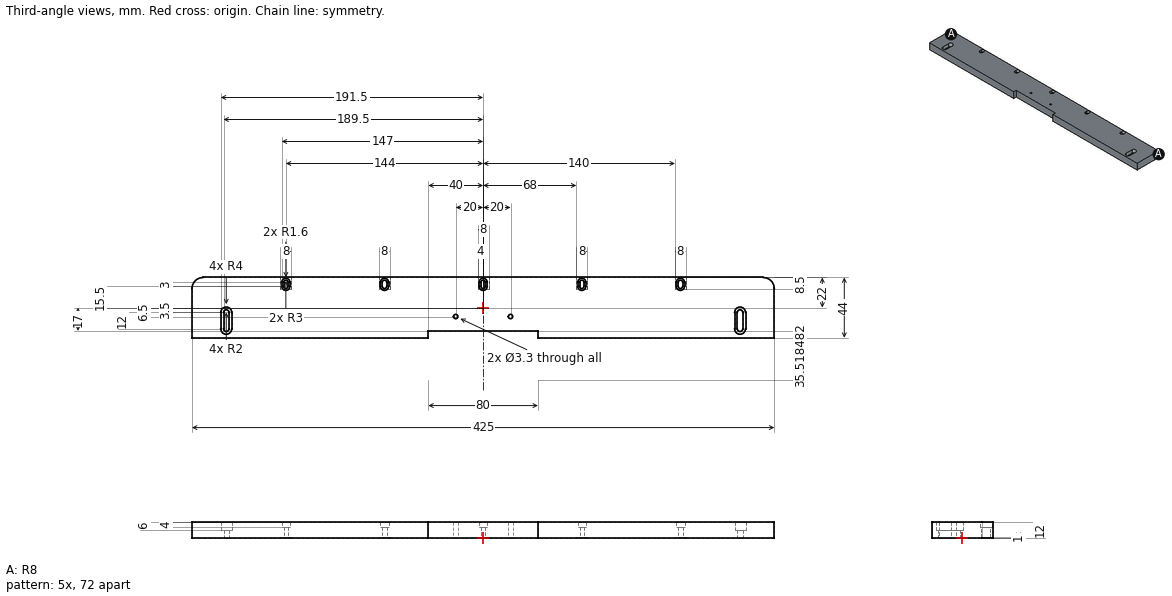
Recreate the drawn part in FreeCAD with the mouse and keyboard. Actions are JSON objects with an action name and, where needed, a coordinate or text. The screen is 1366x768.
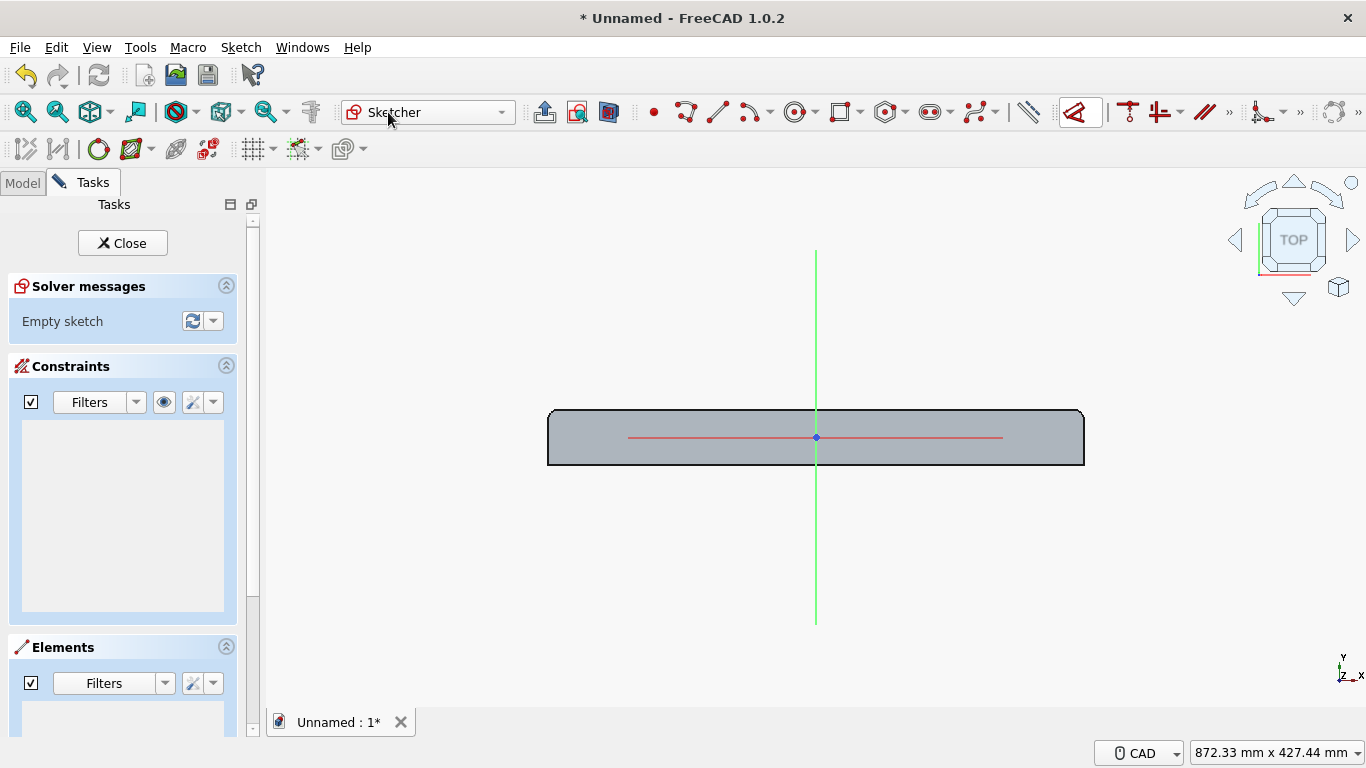
{"action": "left_click", "coordinate": [930, 112]}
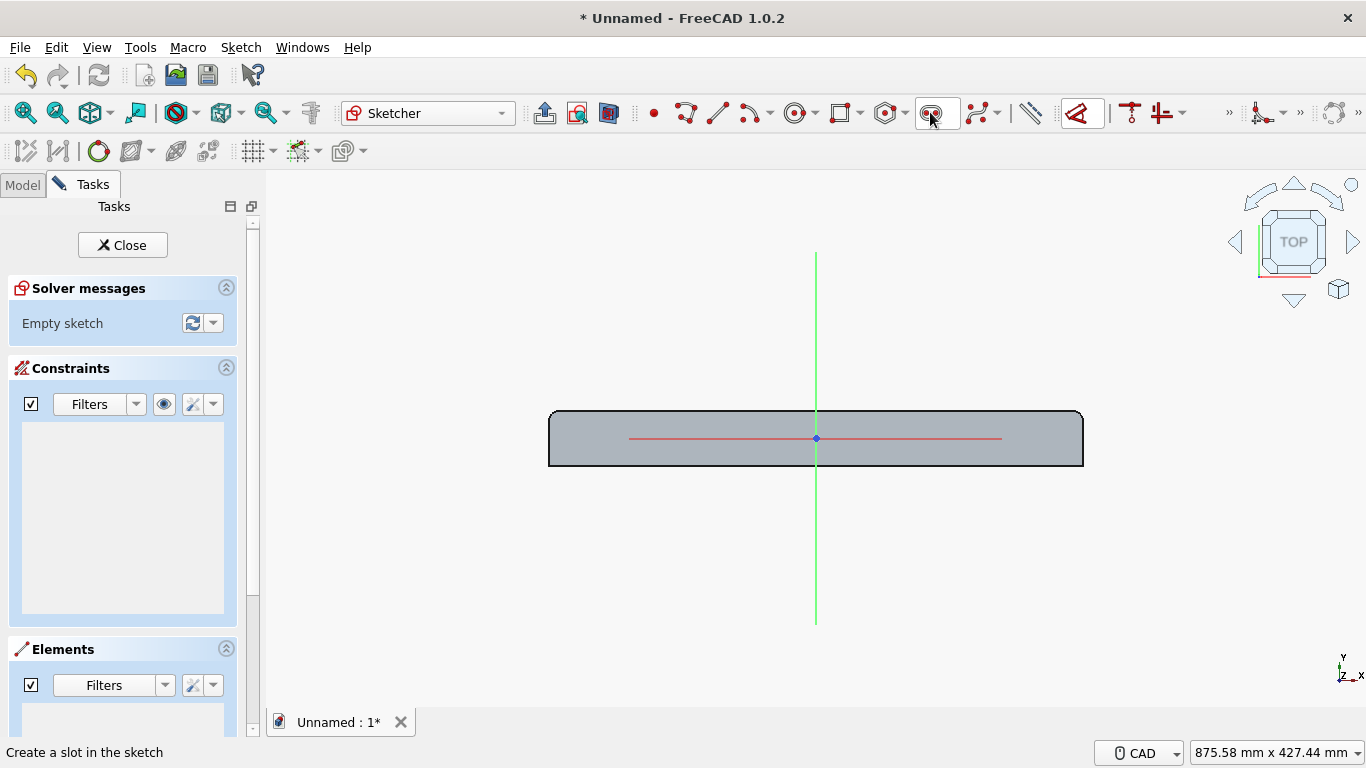
{"action": "scroll", "coordinate": [580, 458], "scroll_direction": "up", "scroll_amount": 8}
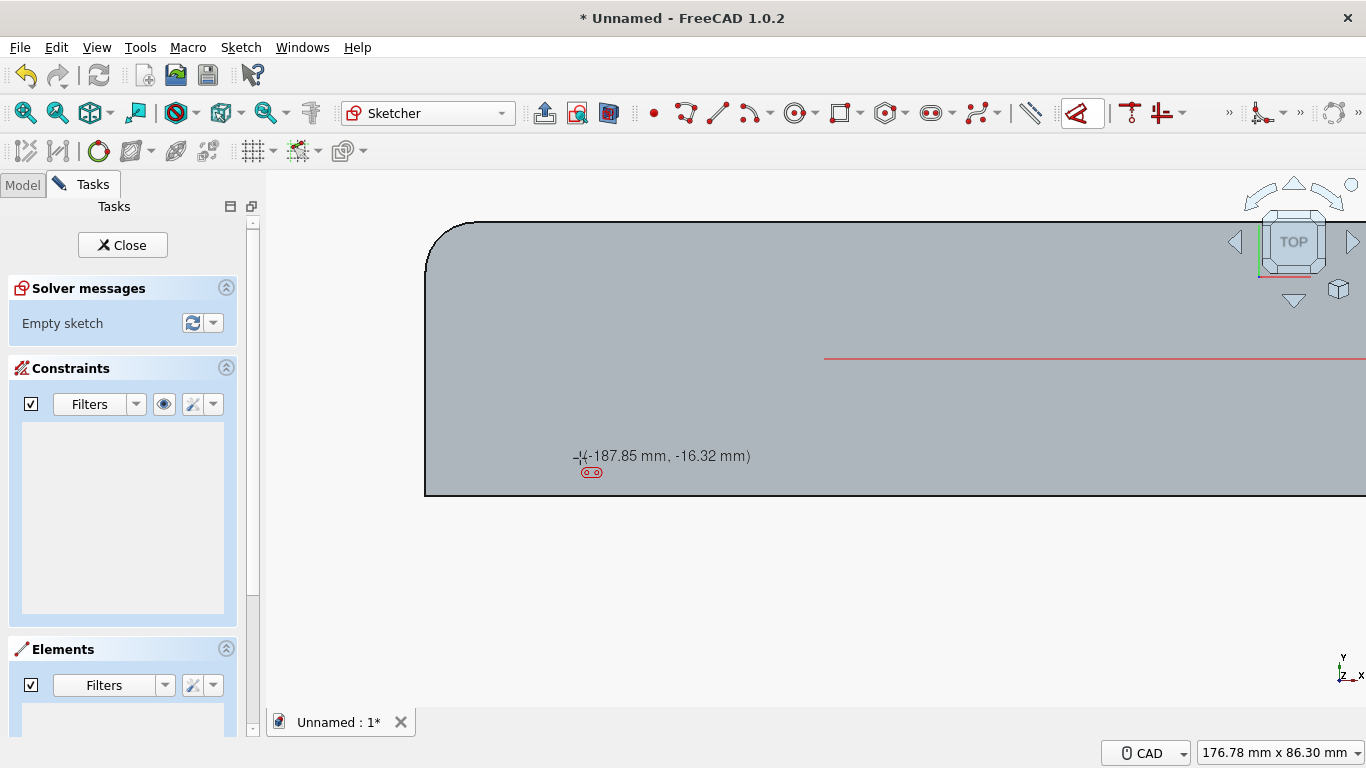
{"action": "scroll", "coordinate": [420, 445], "scroll_direction": "down", "scroll_amount": 7}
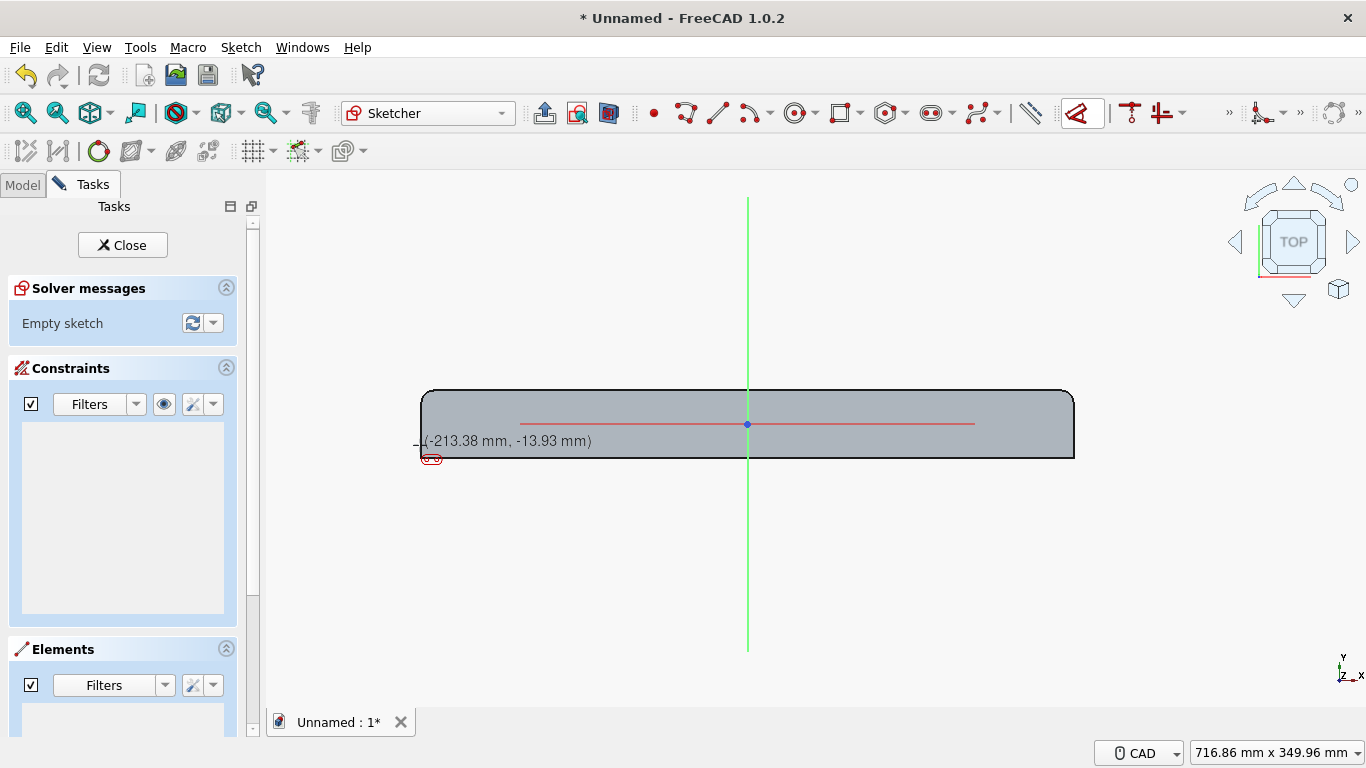
{"action": "left_click", "coordinate": [460, 448]}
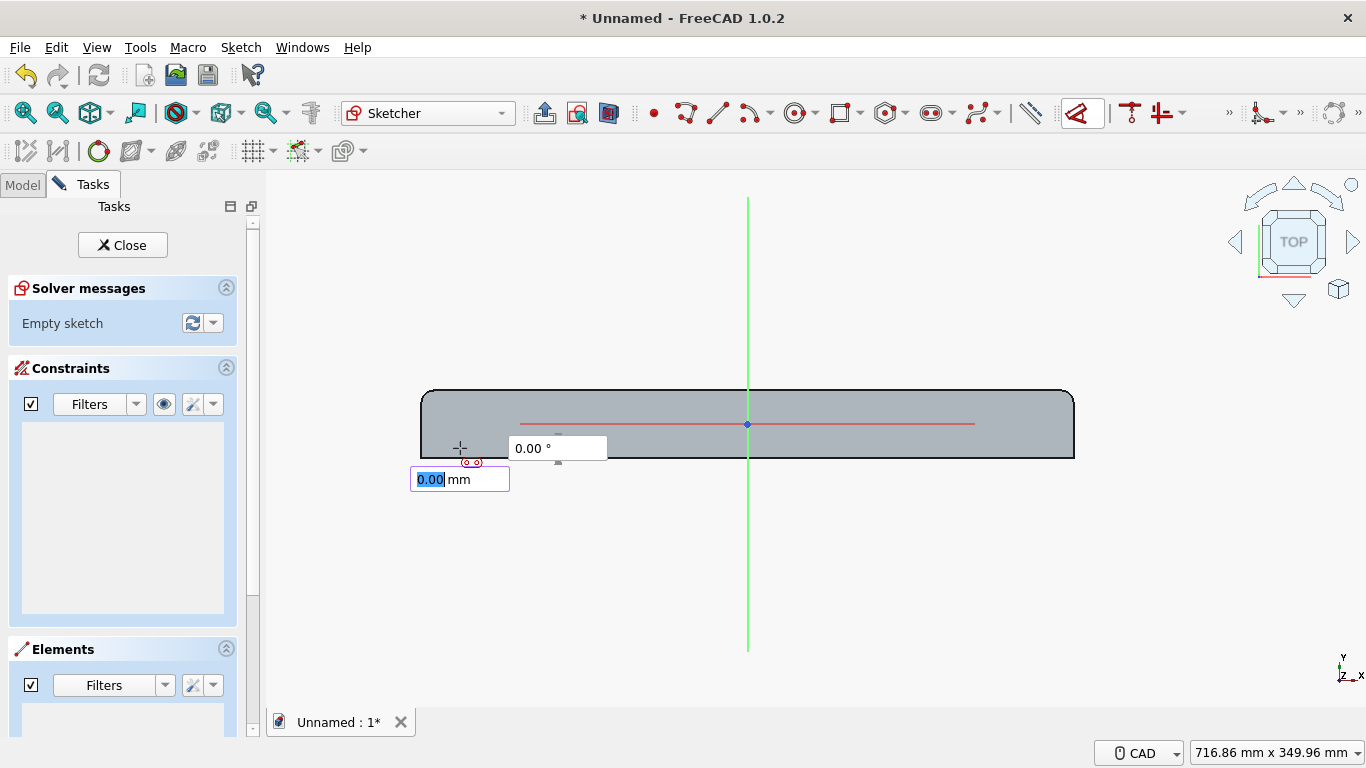
{"action": "scroll", "coordinate": [460, 430], "scroll_direction": "up", "scroll_amount": 6}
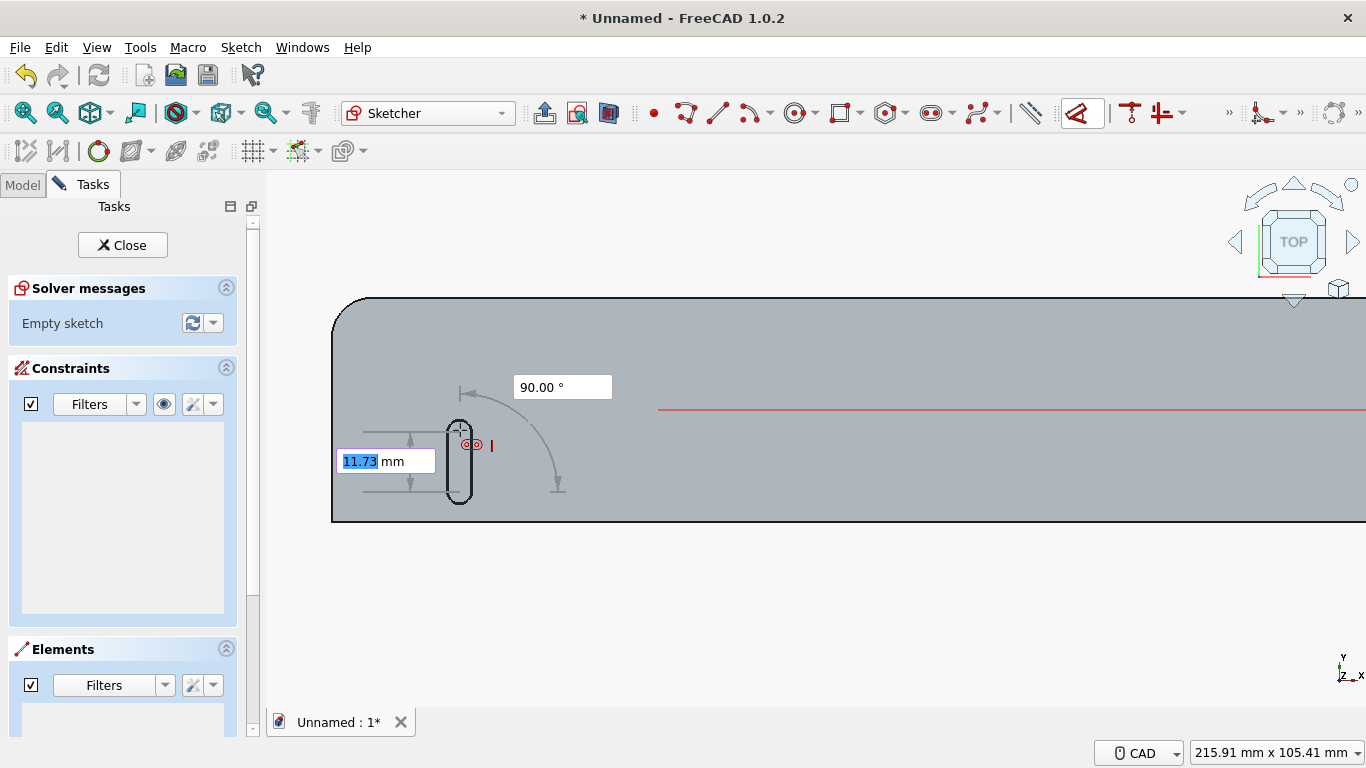
{"action": "left_click", "coordinate": [460, 428]}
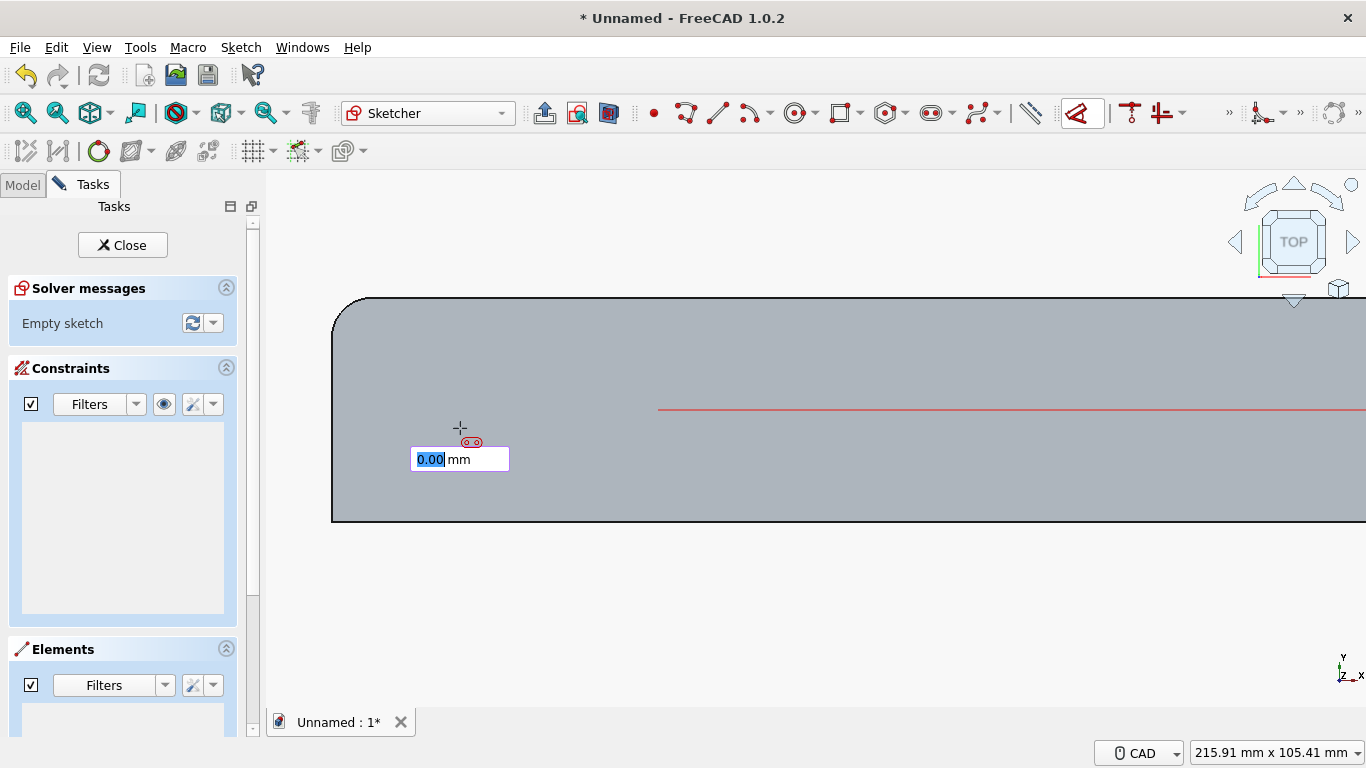
{"action": "left_click", "coordinate": [479, 458]}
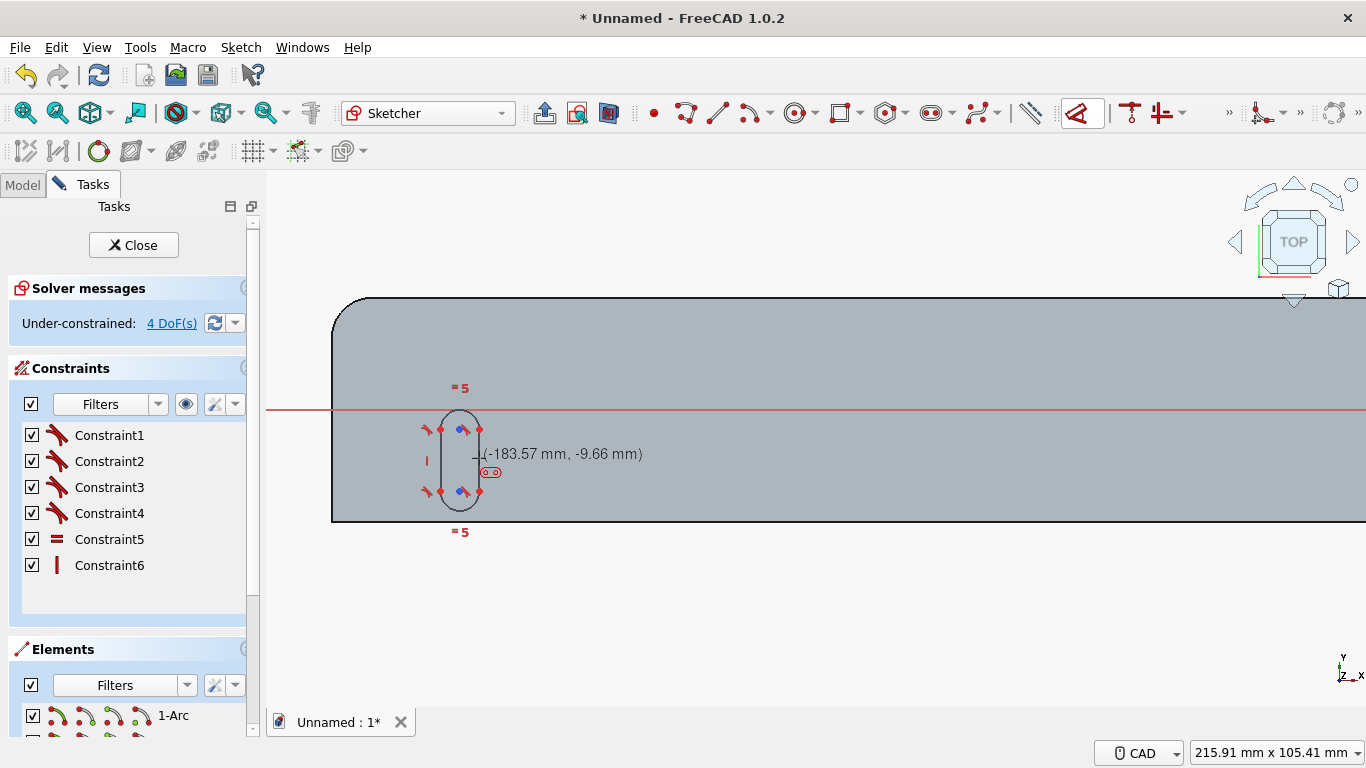
{"action": "scroll", "coordinate": [460, 430], "scroll_direction": "down", "scroll_amount": 6}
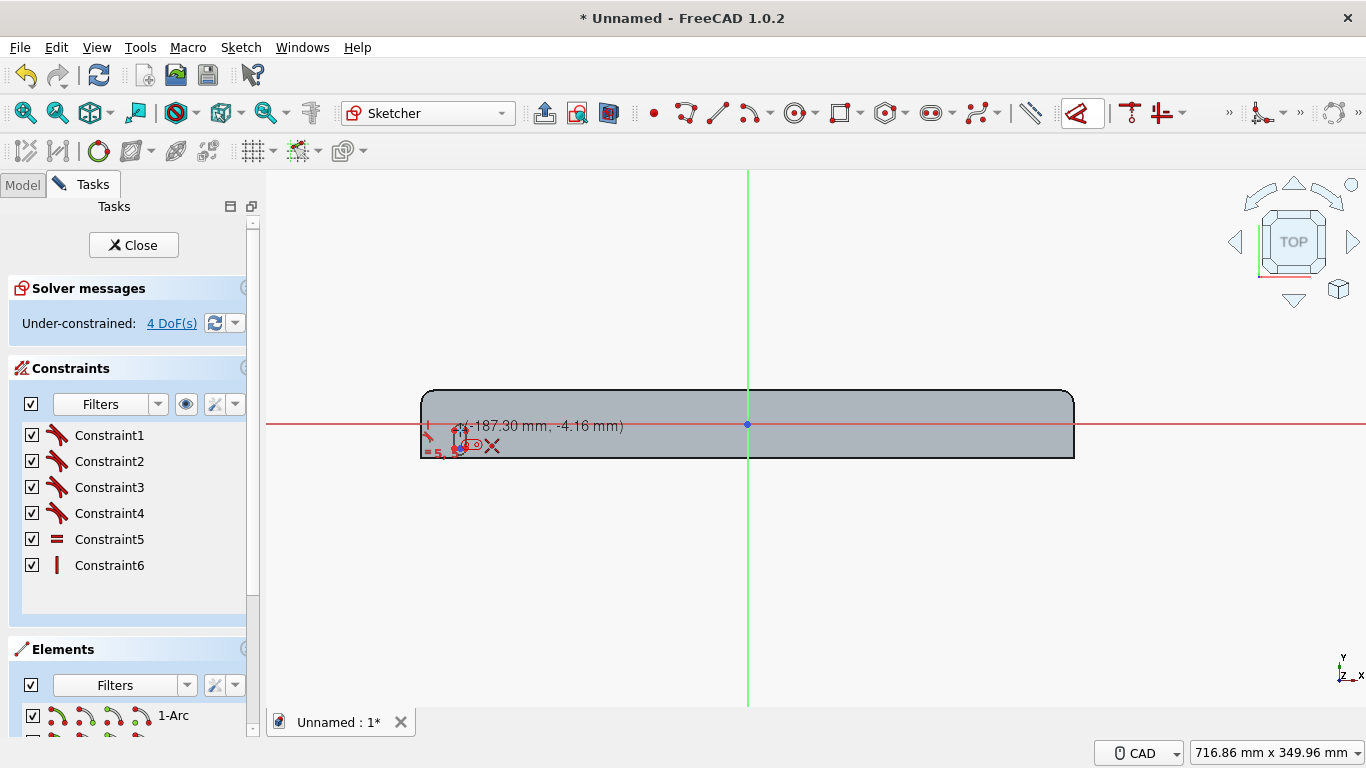
{"action": "scroll", "coordinate": [1035, 448], "scroll_direction": "up", "scroll_amount": 7}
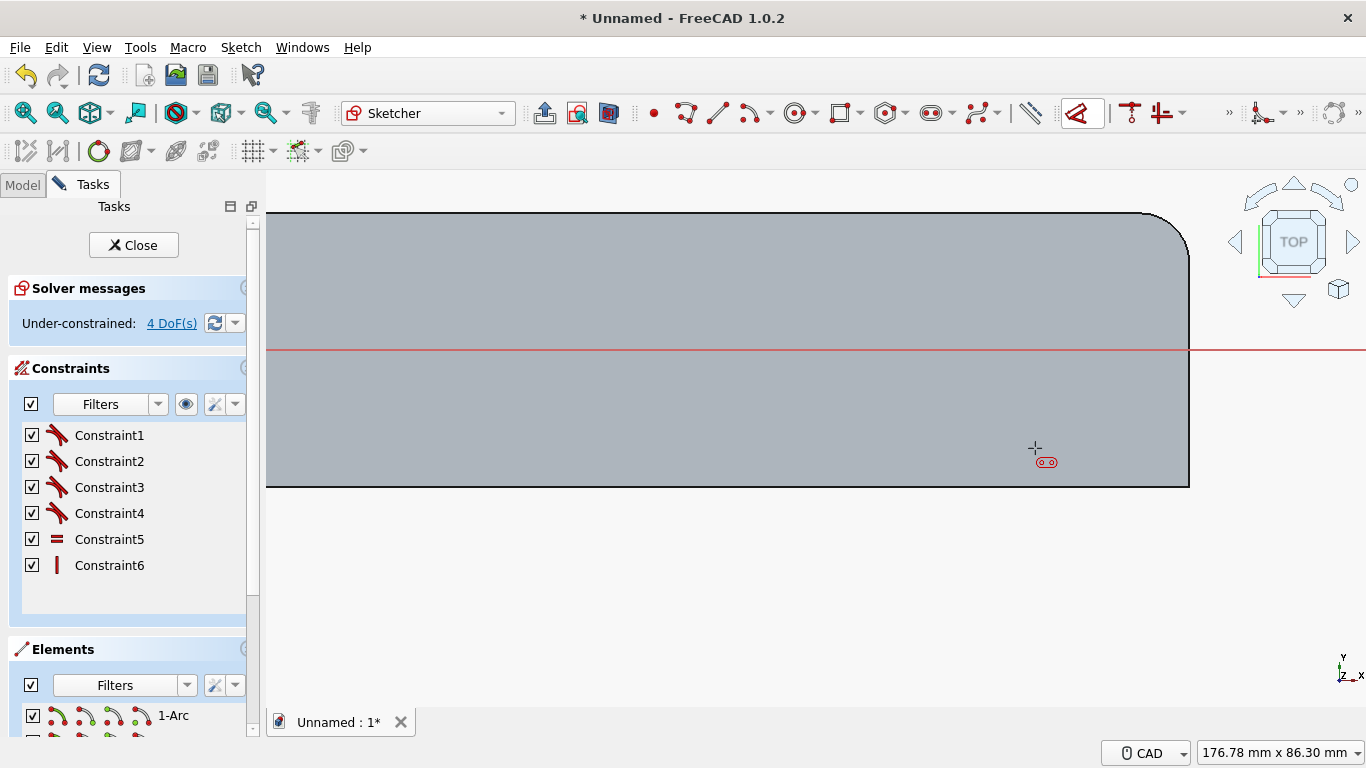
{"action": "scroll", "coordinate": [1036, 448], "scroll_direction": "down", "scroll_amount": 7}